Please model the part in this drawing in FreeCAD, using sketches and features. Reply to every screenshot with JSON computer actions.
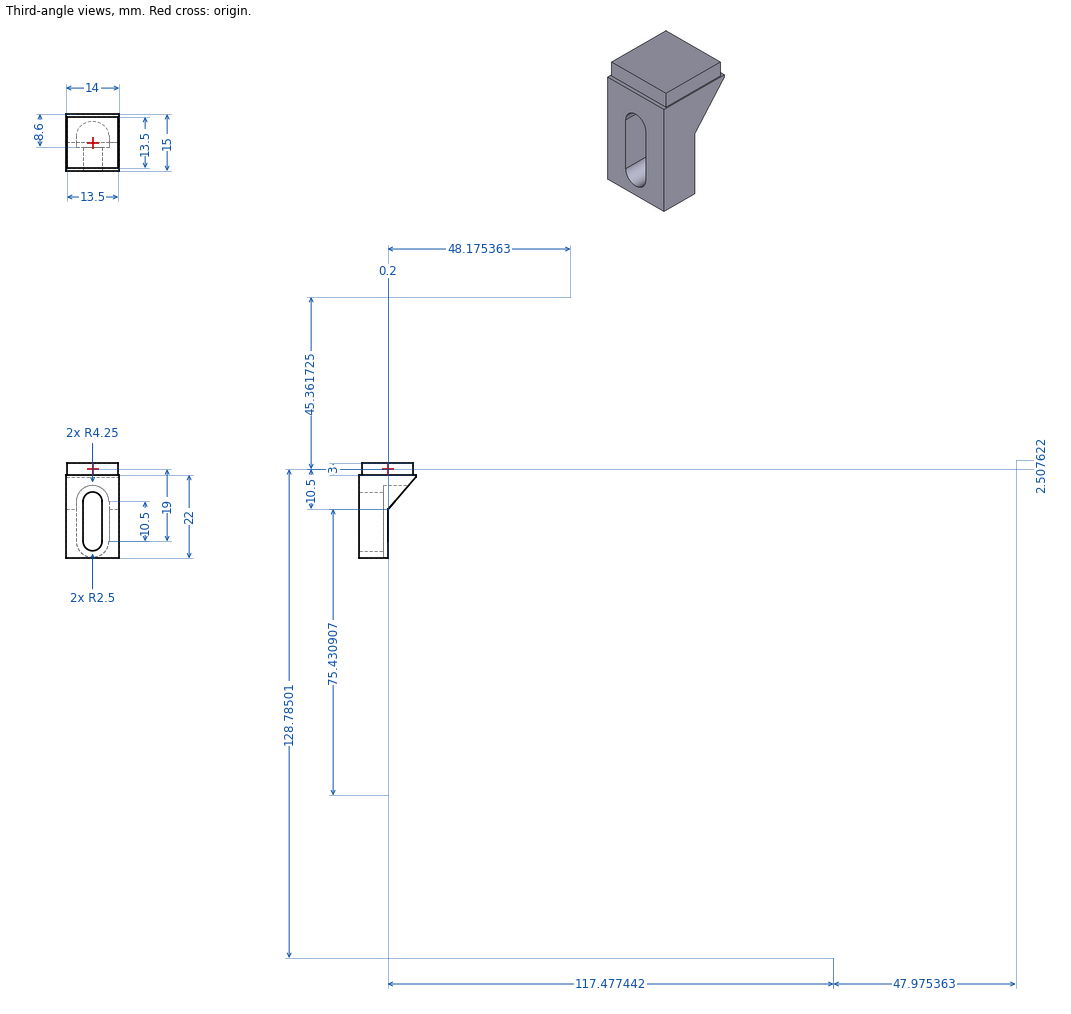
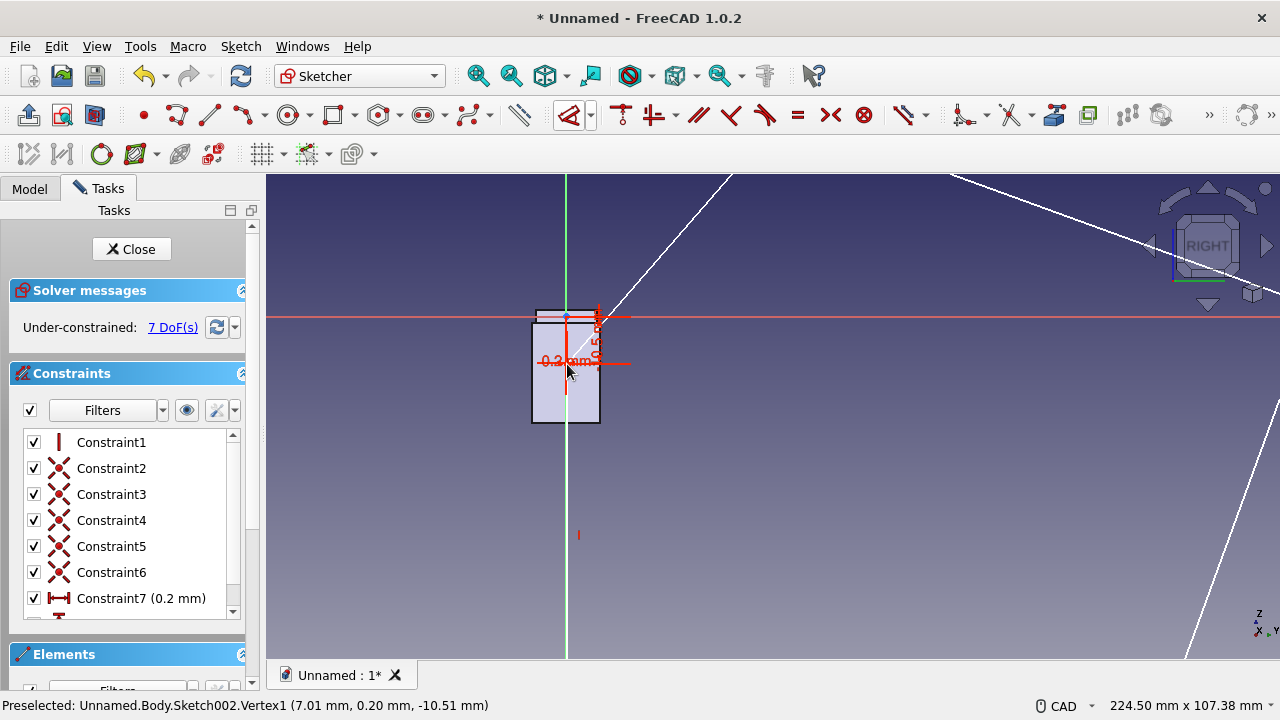
{"action": "left_click", "coordinate": [567, 466]}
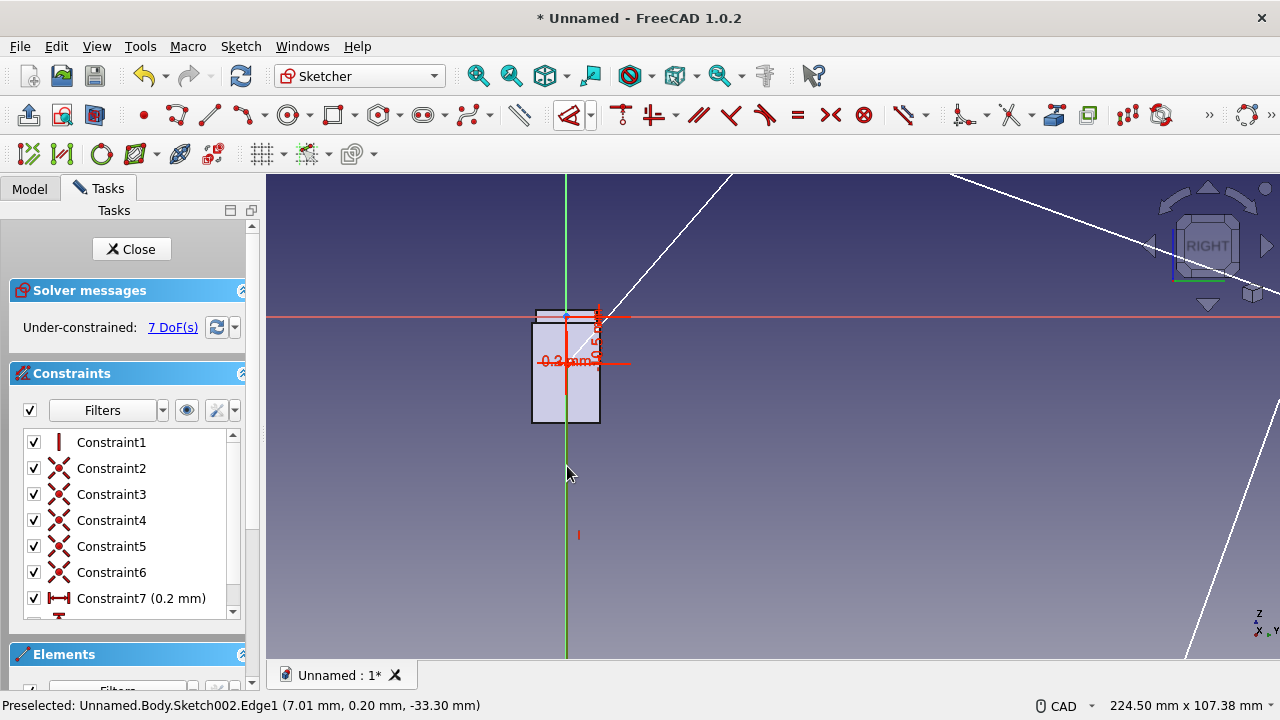
{"action": "left_click", "coordinate": [590, 116]}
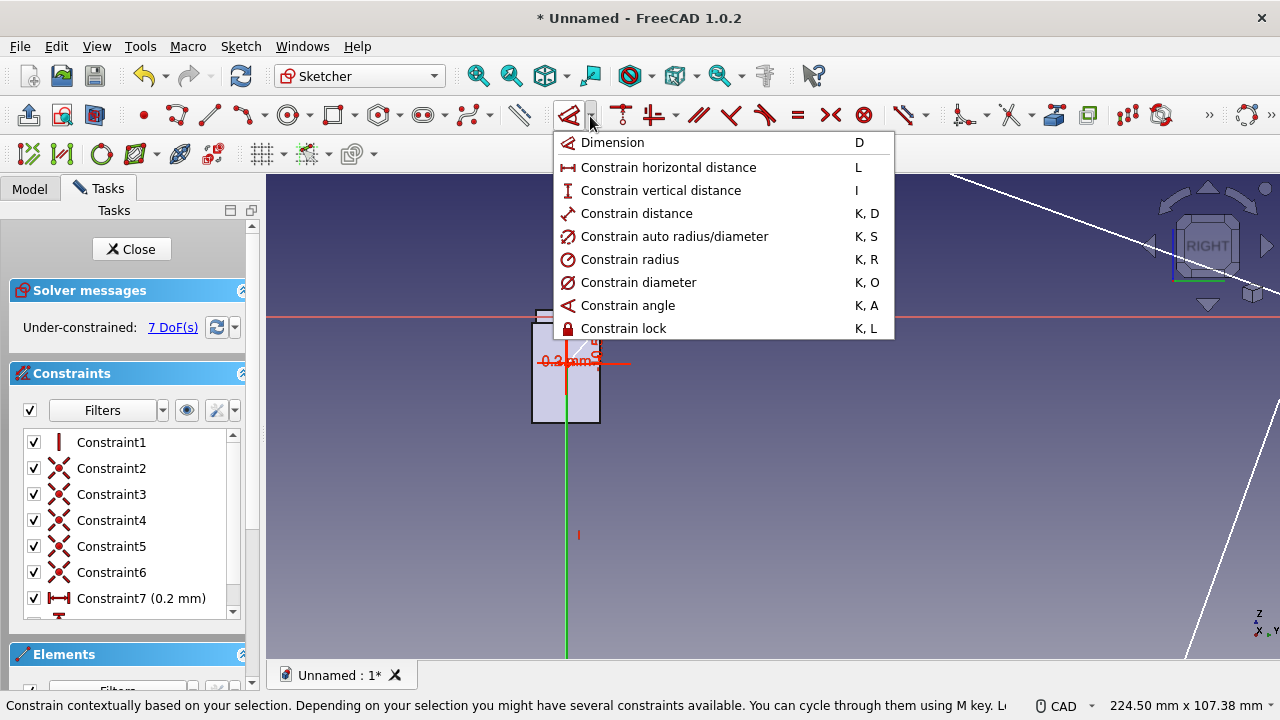
{"action": "left_click", "coordinate": [724, 190]}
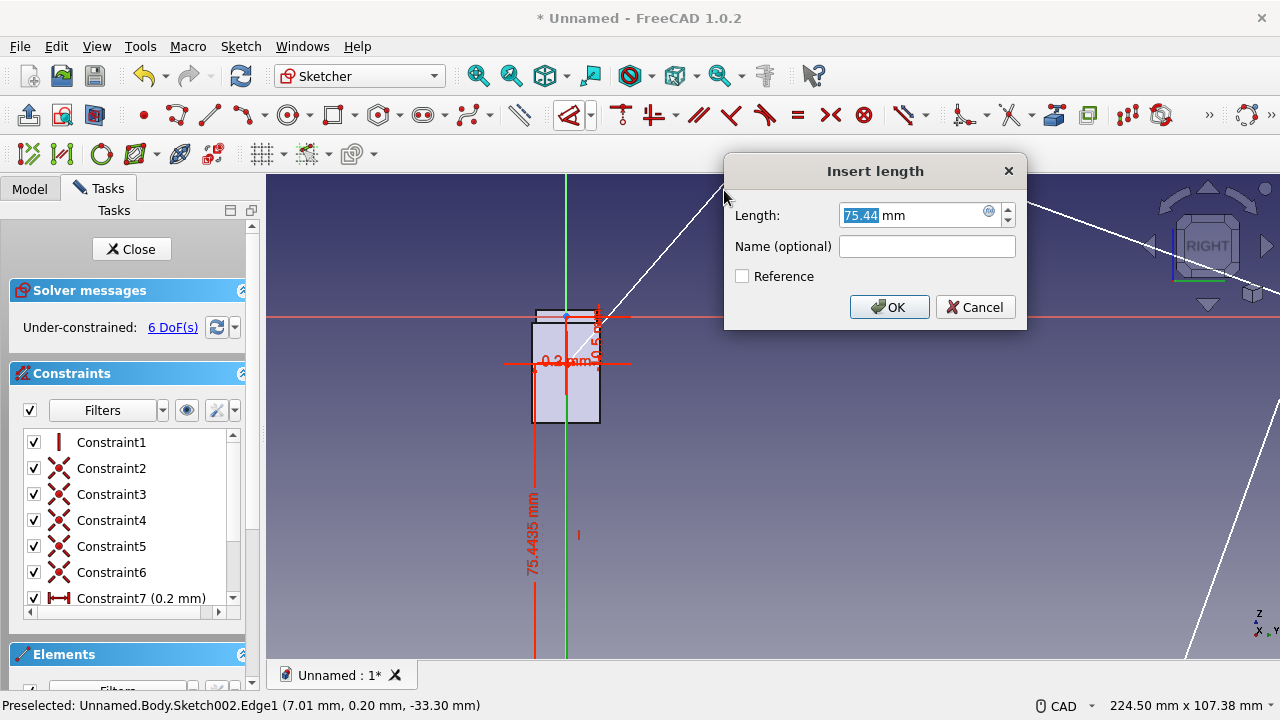
{"action": "type", "text": "75.430907"}
{"action": "key", "text": "Return"}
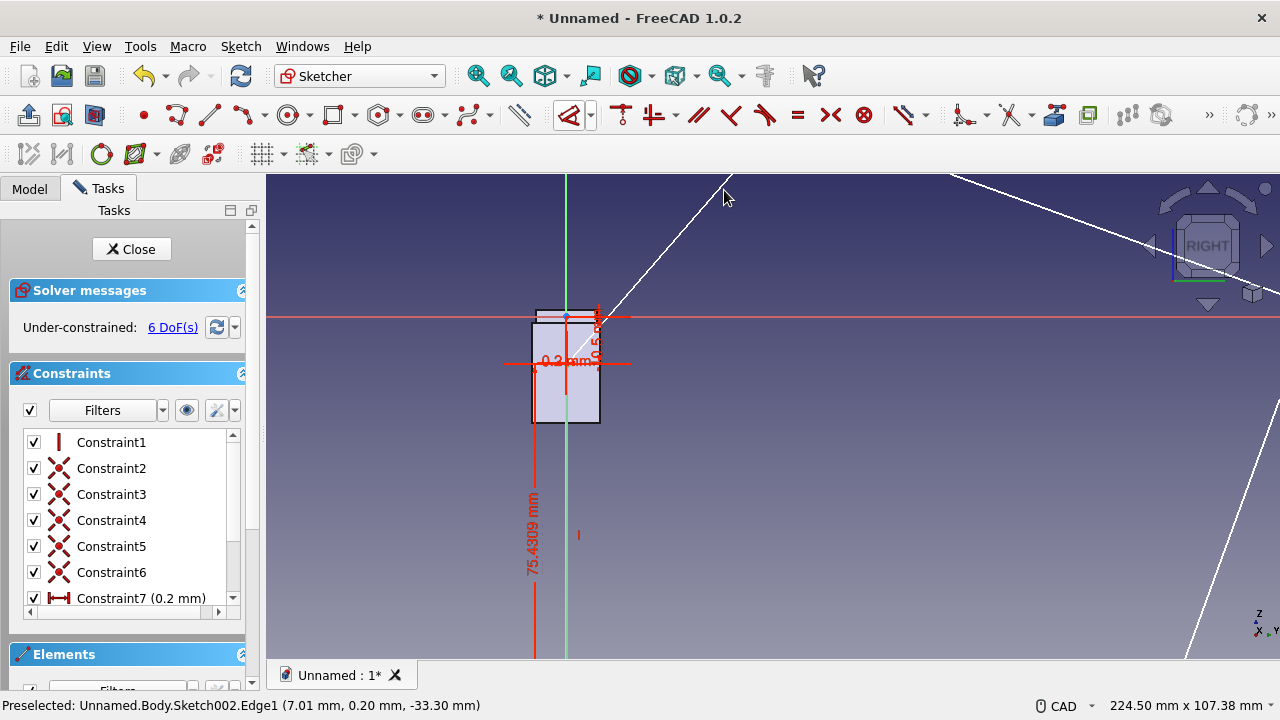
{"action": "scroll", "coordinate": [568, 365], "scroll_direction": "down", "scroll_amount": 5}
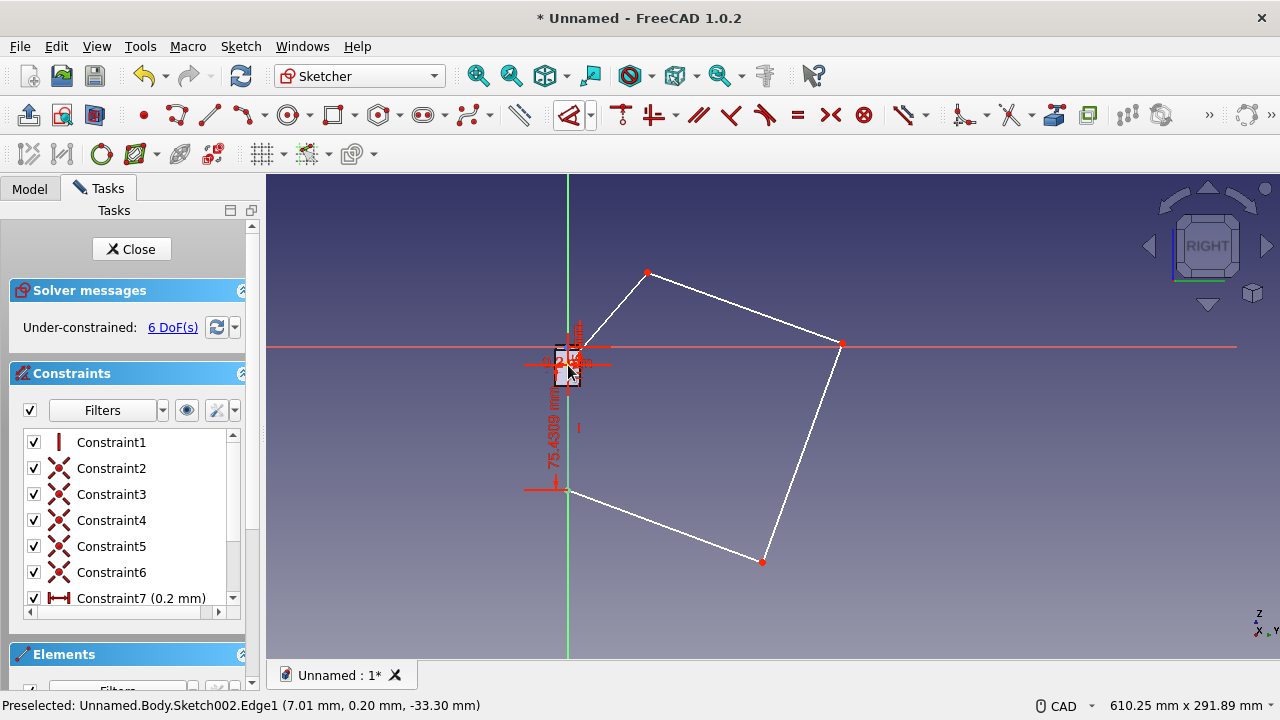
{"action": "scroll", "coordinate": [843, 344], "scroll_direction": "up", "scroll_amount": 12}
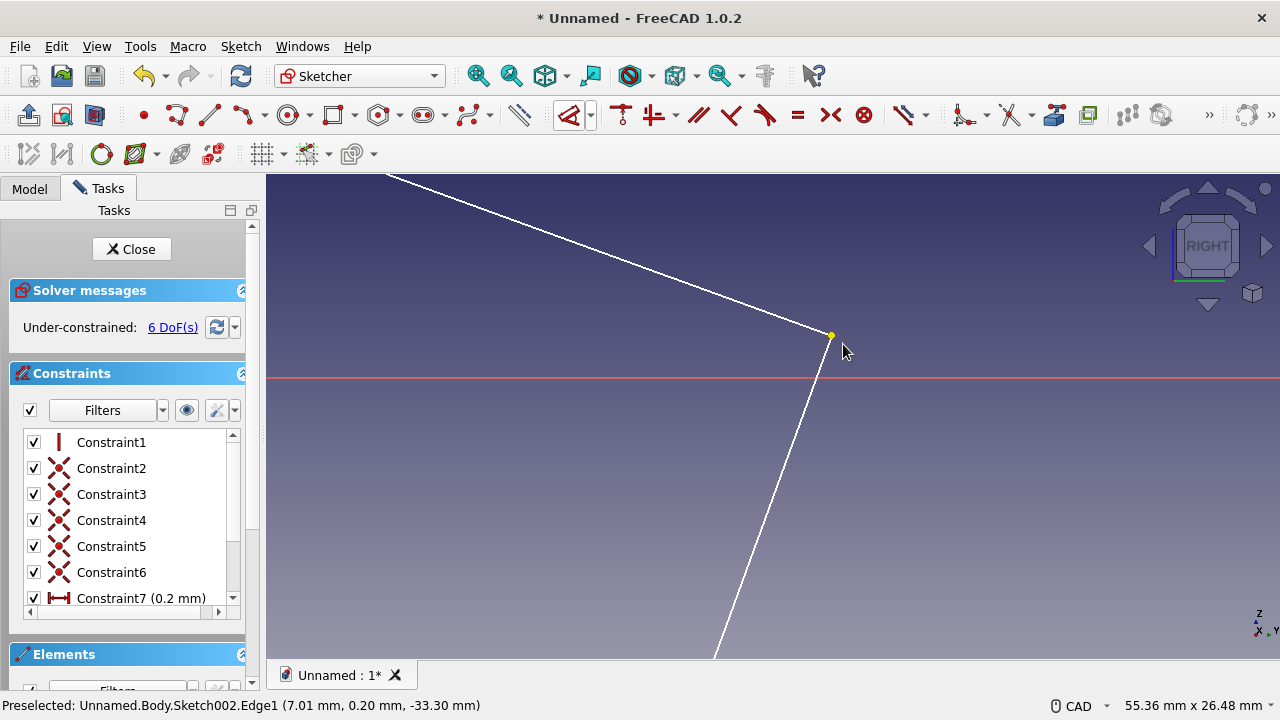
{"action": "left_click", "coordinate": [832, 336]}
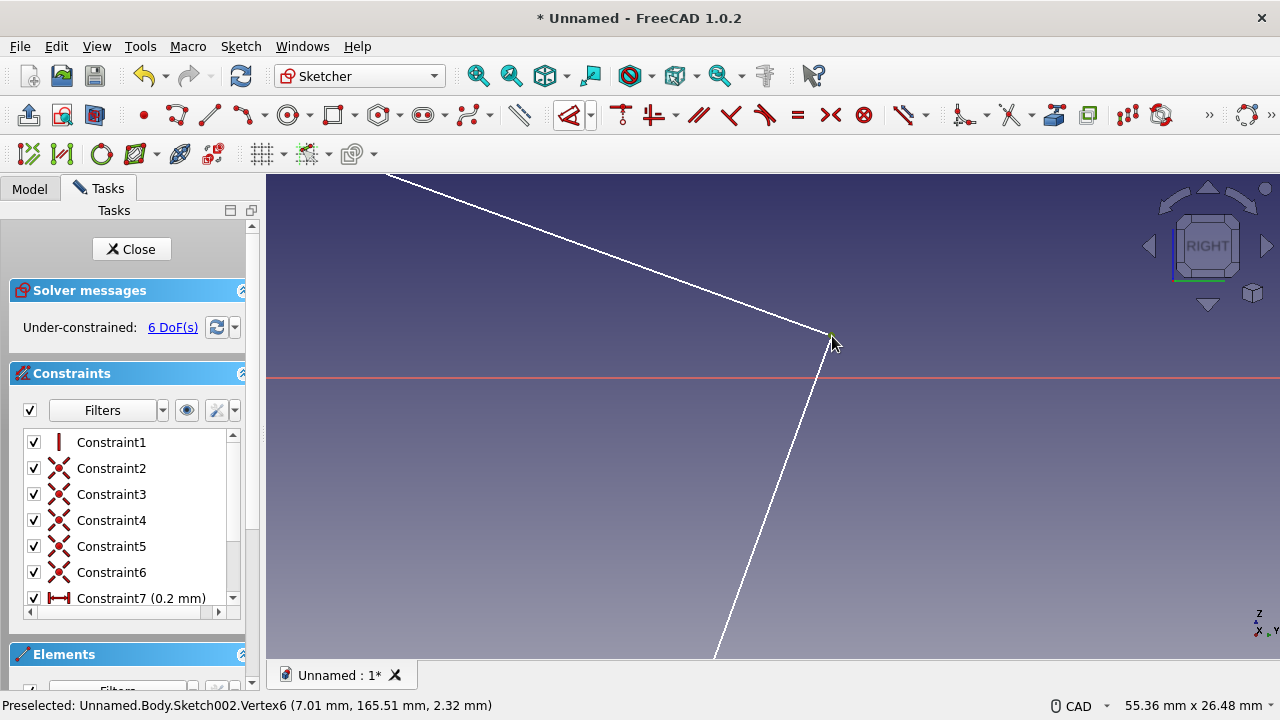
{"action": "key", "text": "i"}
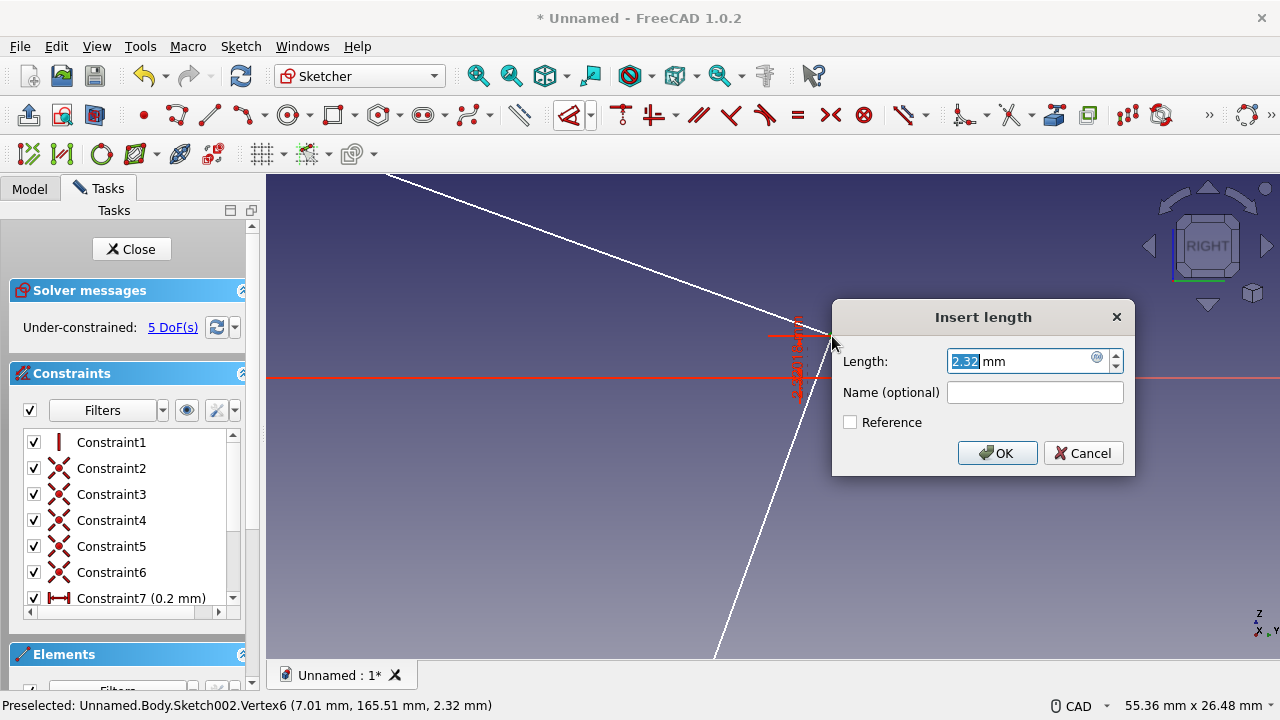
{"action": "type", "text": "2.507622"}
{"action": "key", "text": "Return"}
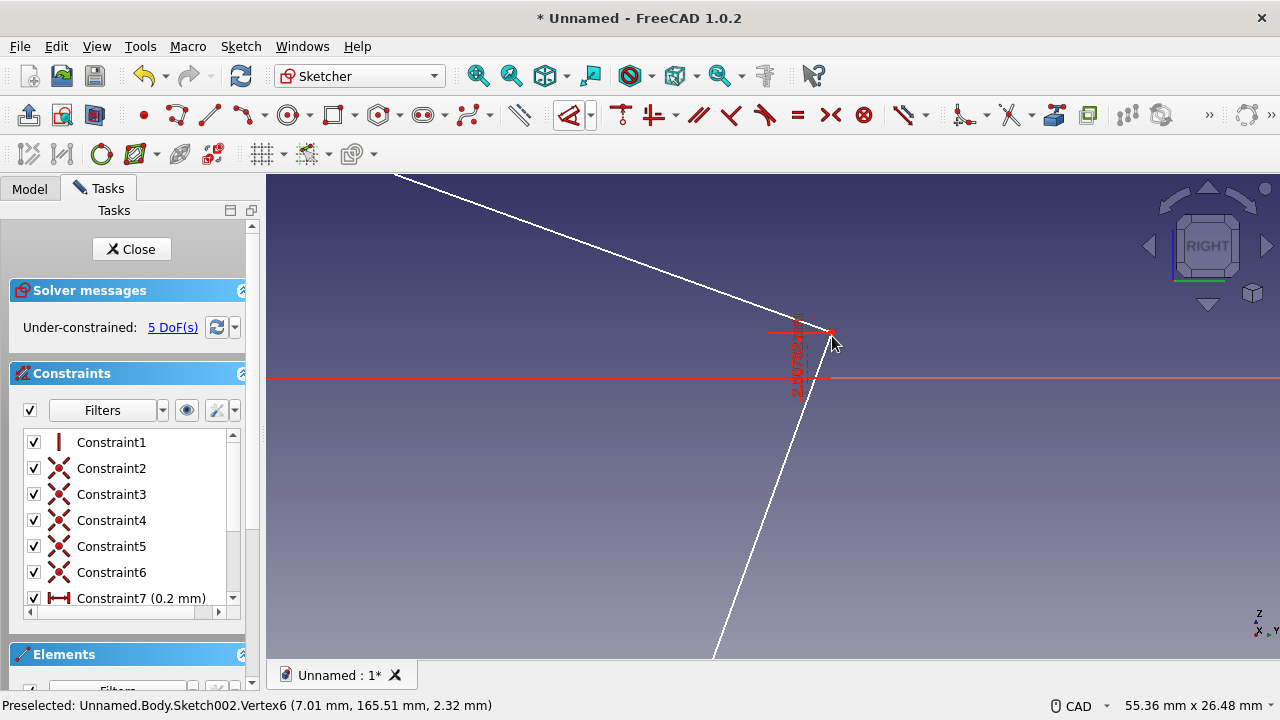
{"action": "scroll", "coordinate": [843, 344], "scroll_direction": "down", "scroll_amount": 12}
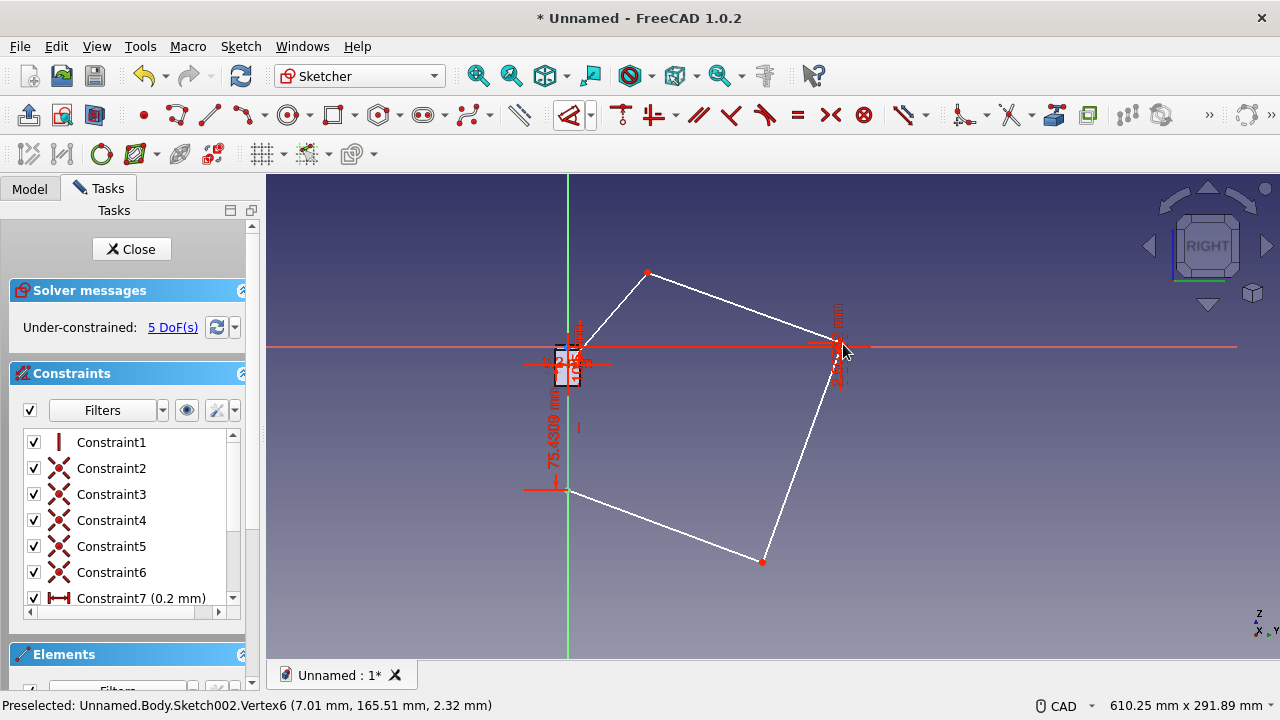
{"action": "left_click", "coordinate": [763, 563]}